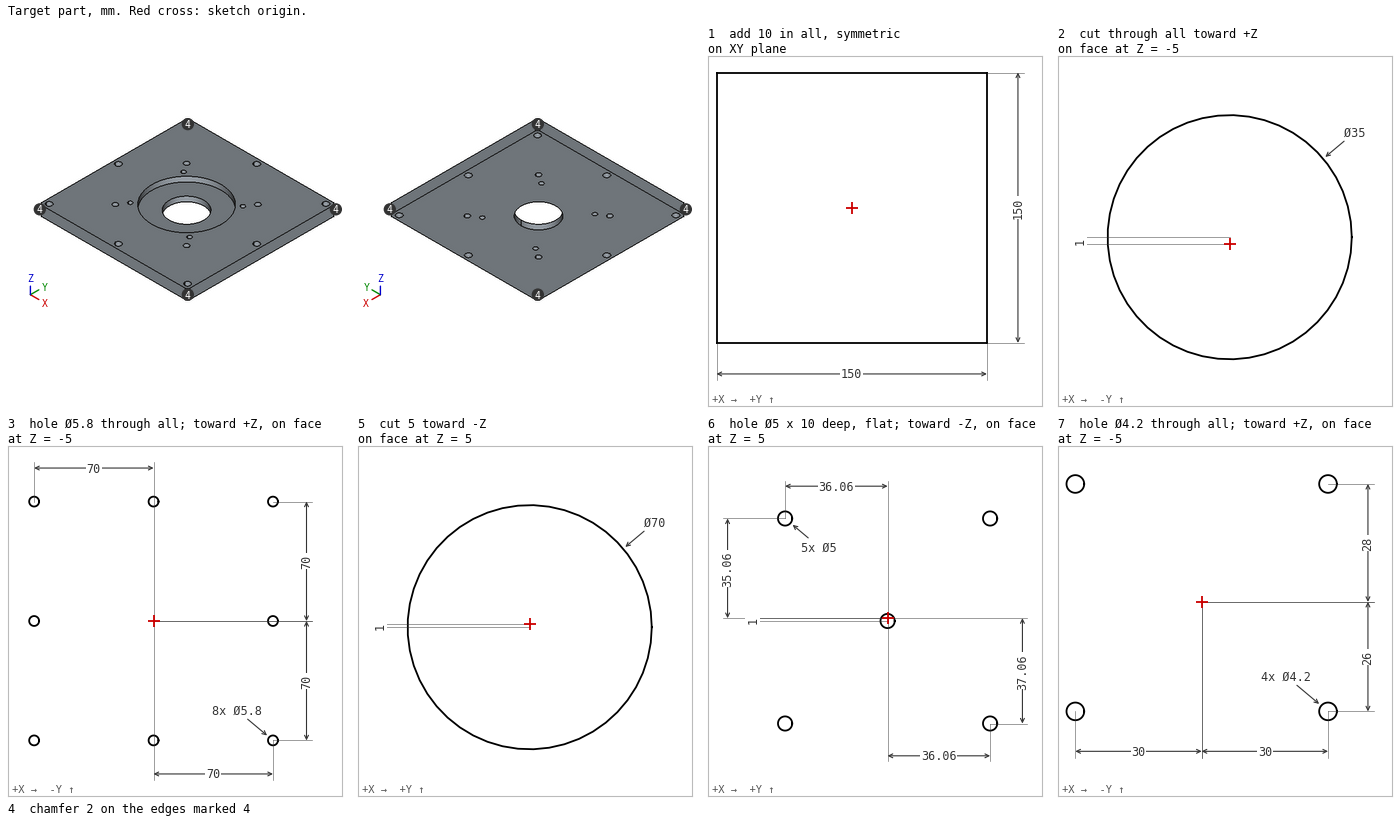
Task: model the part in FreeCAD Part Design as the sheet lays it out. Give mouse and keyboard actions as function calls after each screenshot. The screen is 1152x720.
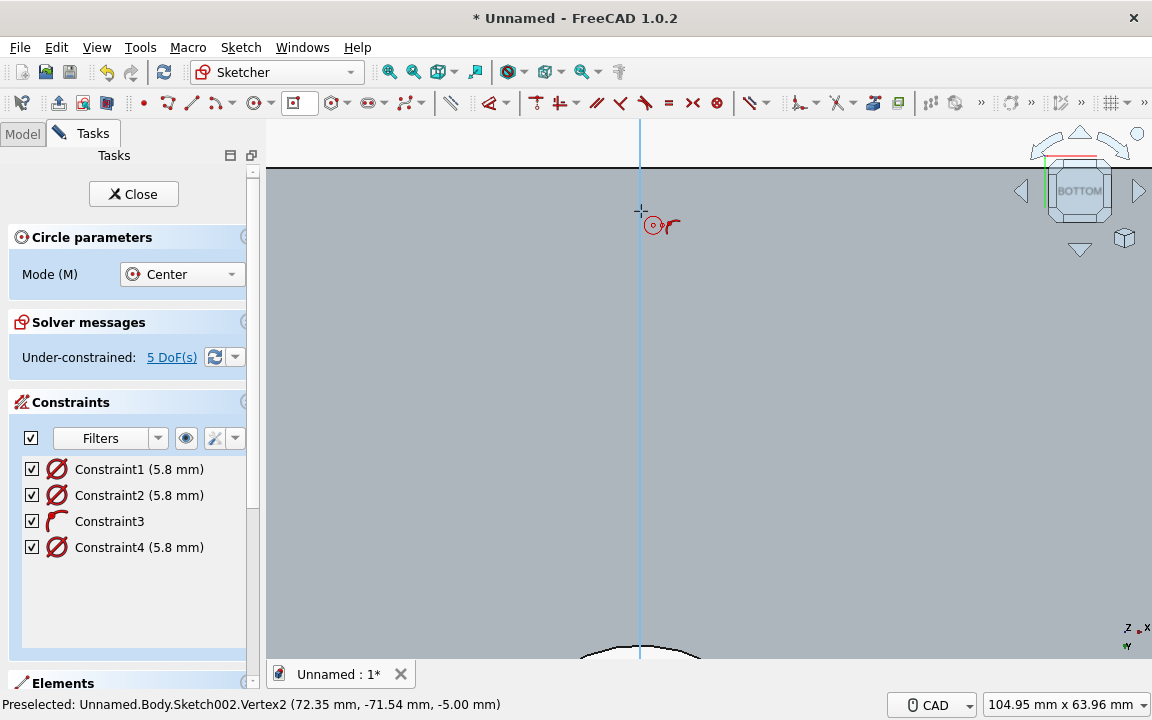
click(640, 211)
move(658, 193)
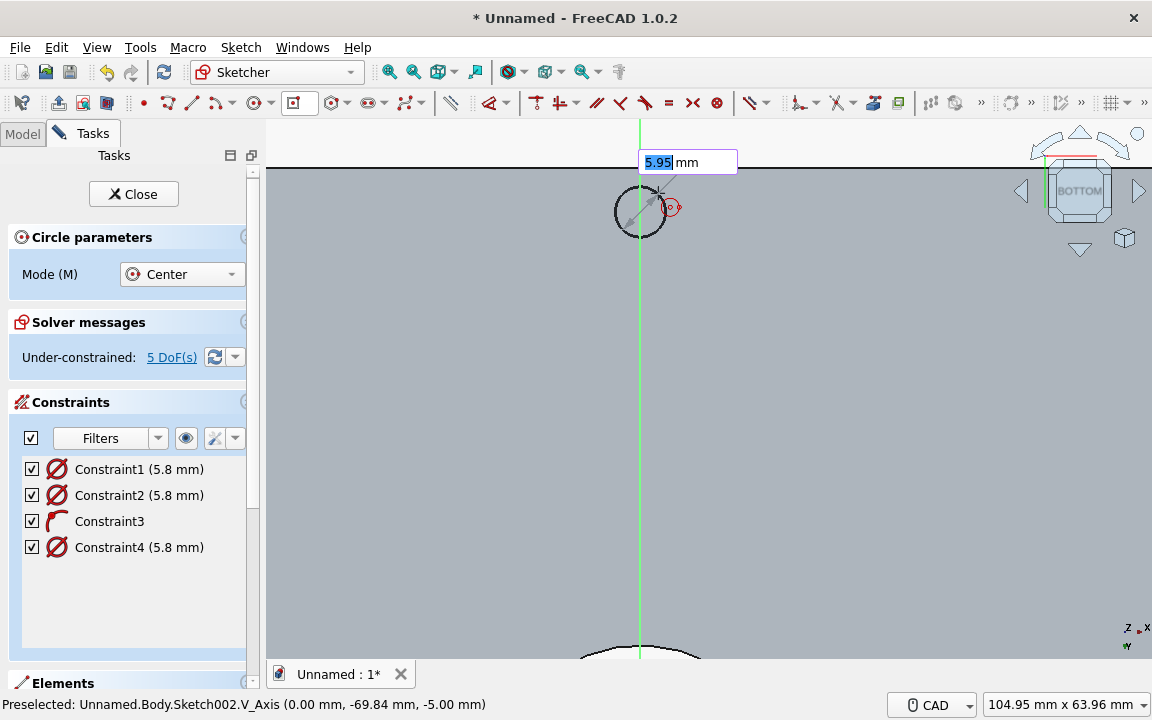
text(5.8)
key(Return)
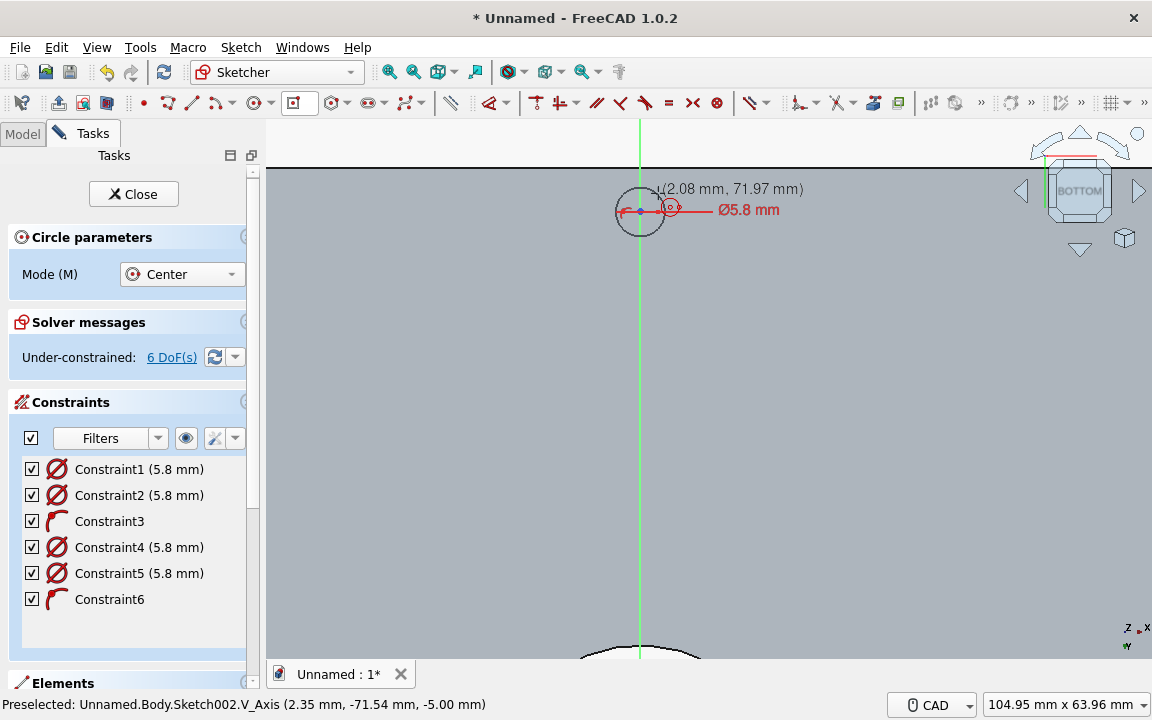
scroll(641, 211, down, 6)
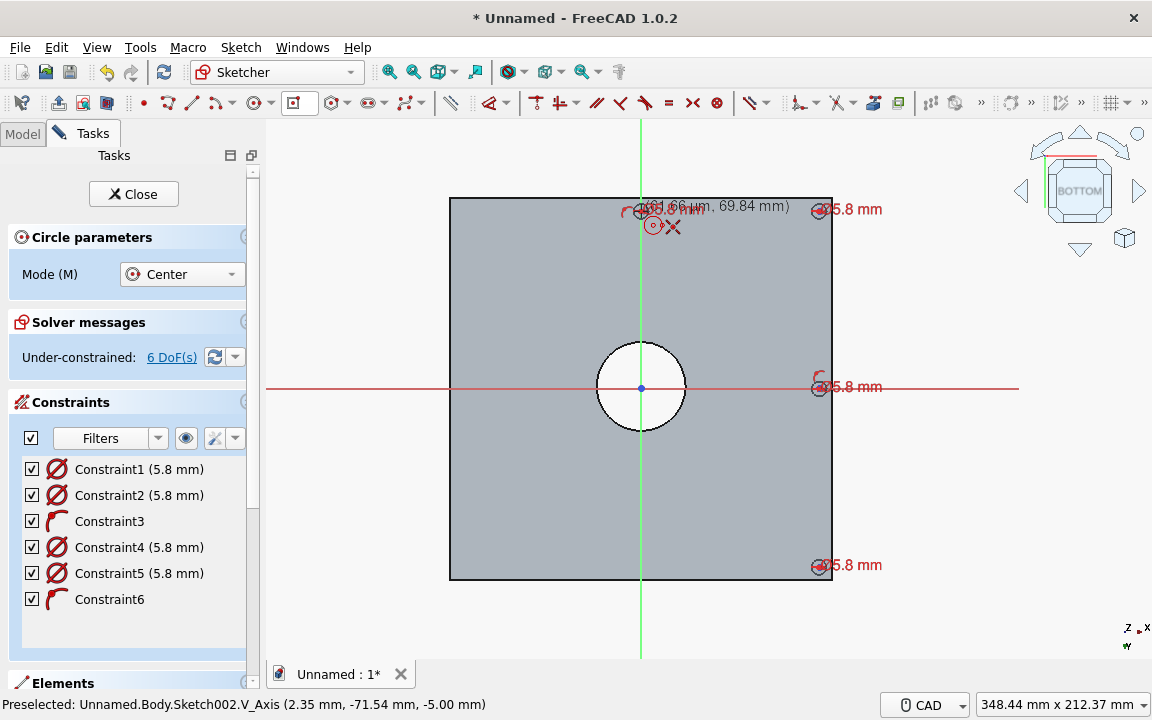
scroll(463, 211, up, 6)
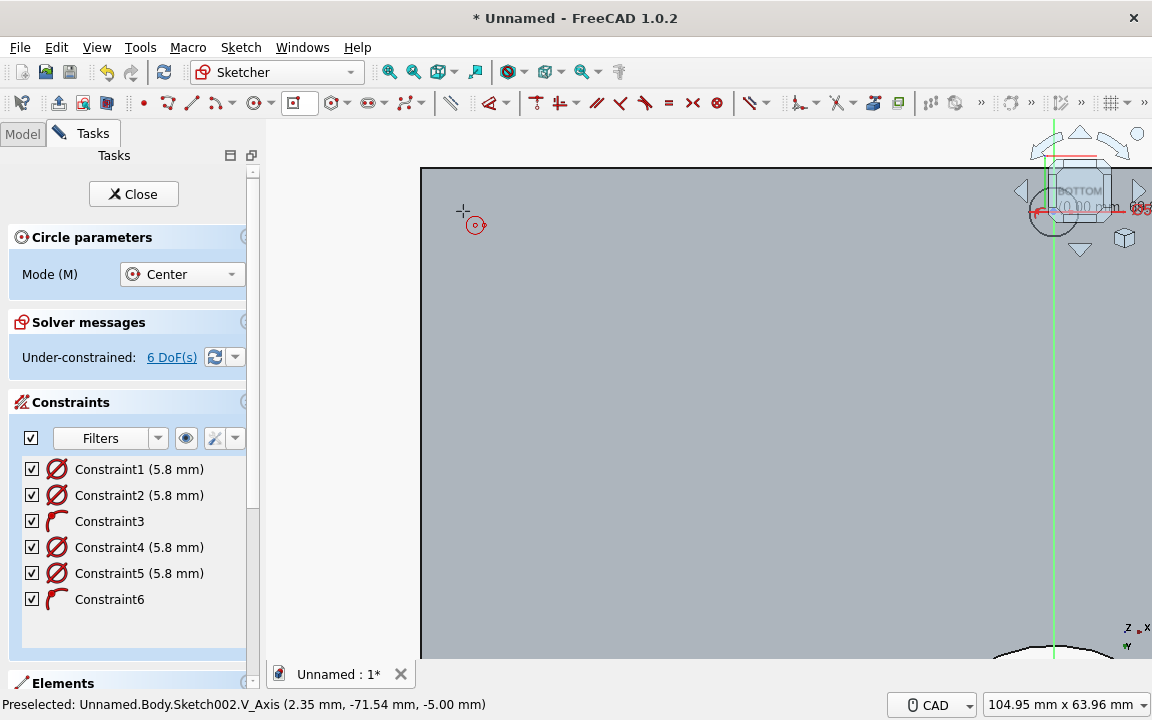
click(463, 211)
move(480, 193)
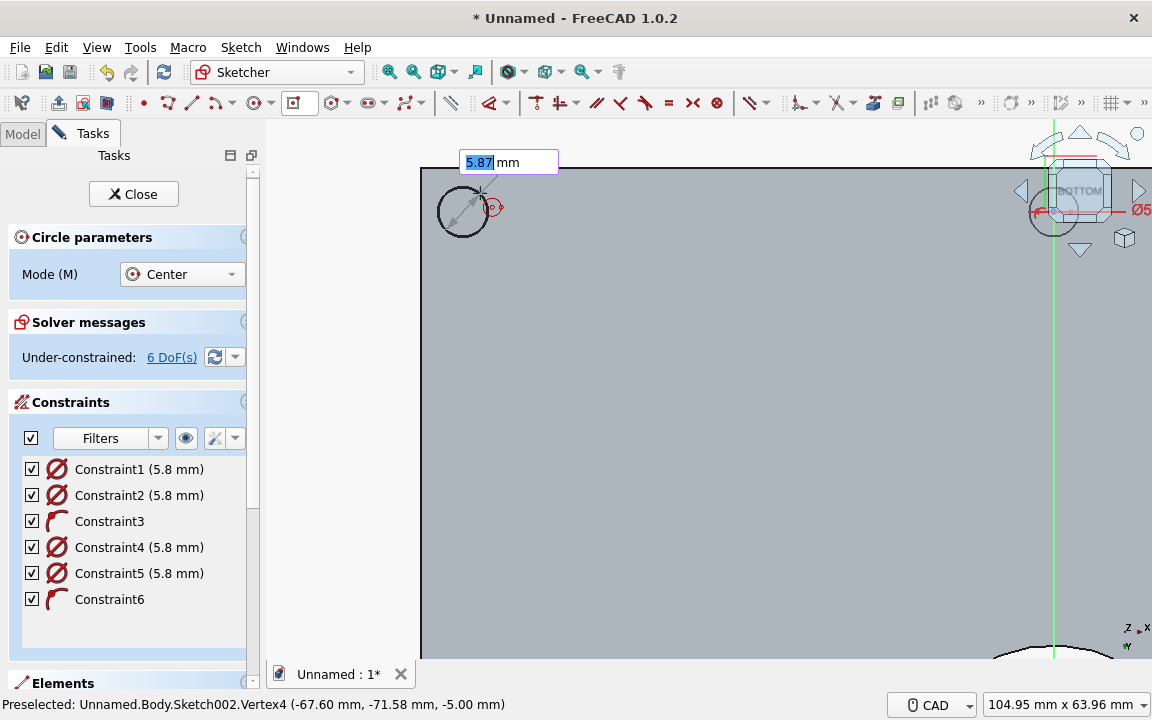
text(5.8)
key(Return)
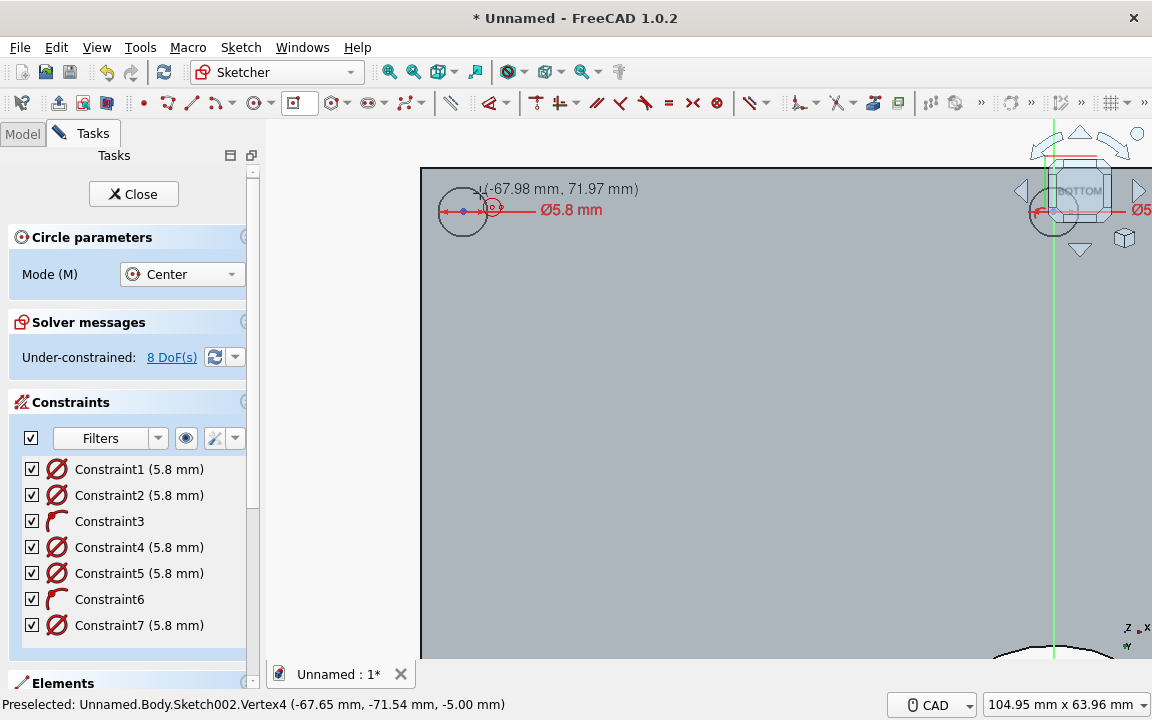
scroll(462, 211, down, 6)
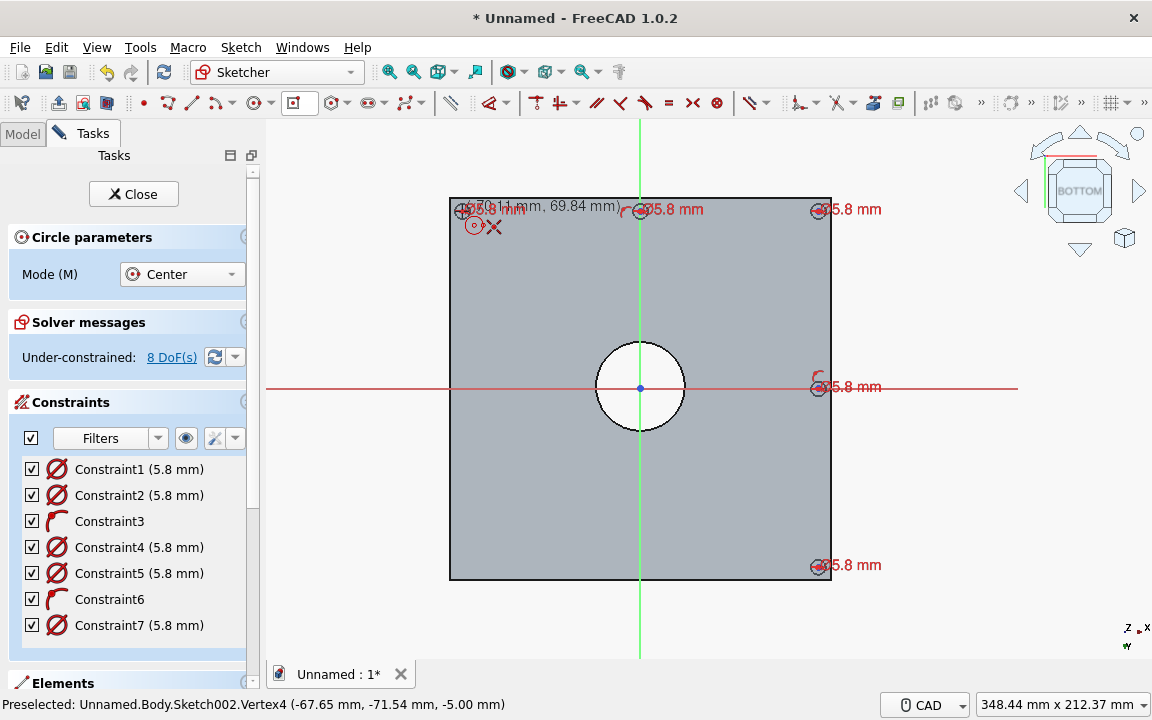
scroll(462, 389, up, 6)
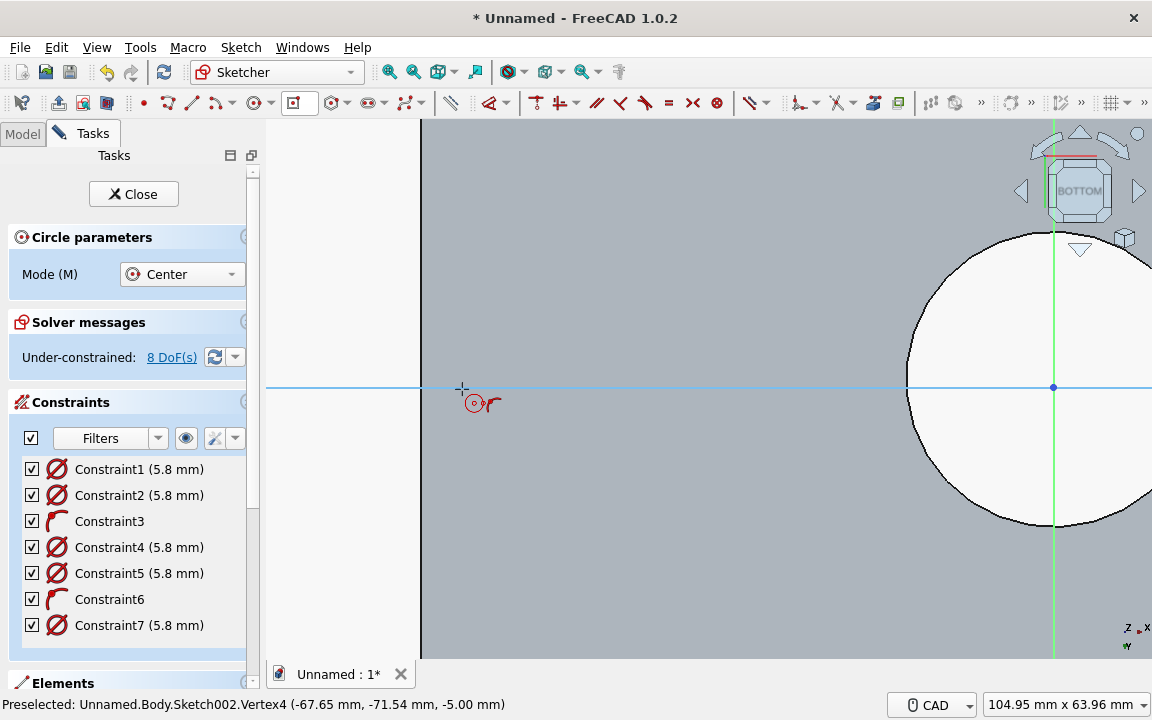
click(463, 388)
move(480, 371)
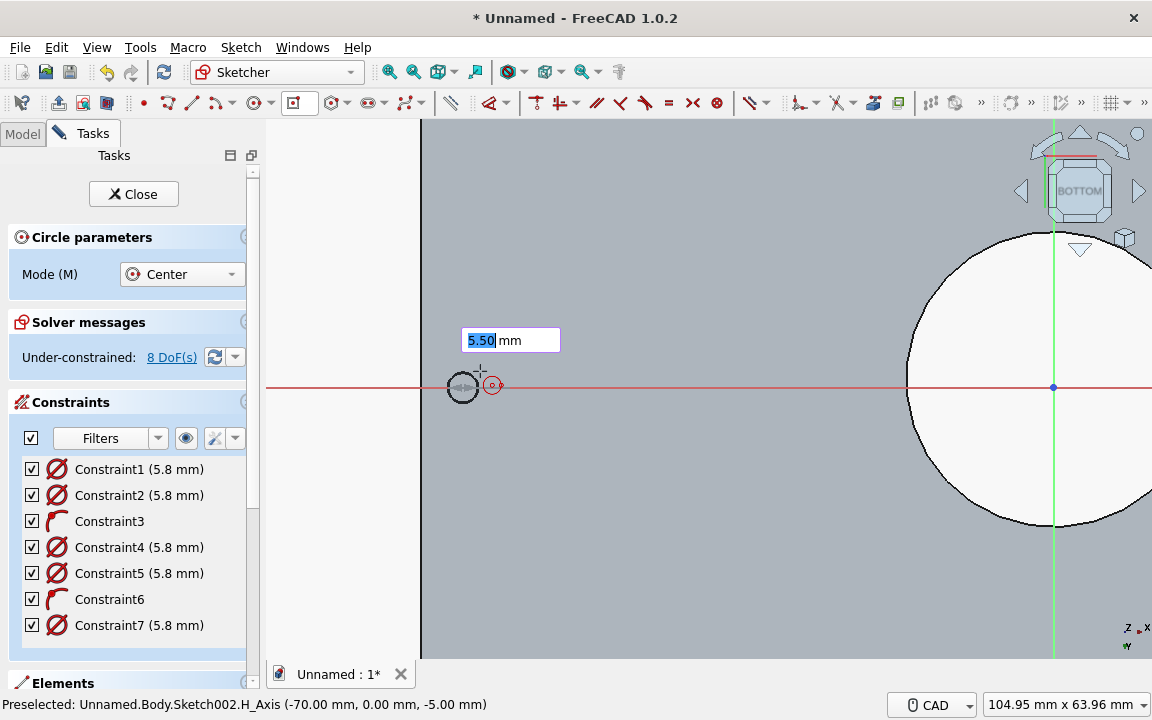
text(5.8)
key(Return)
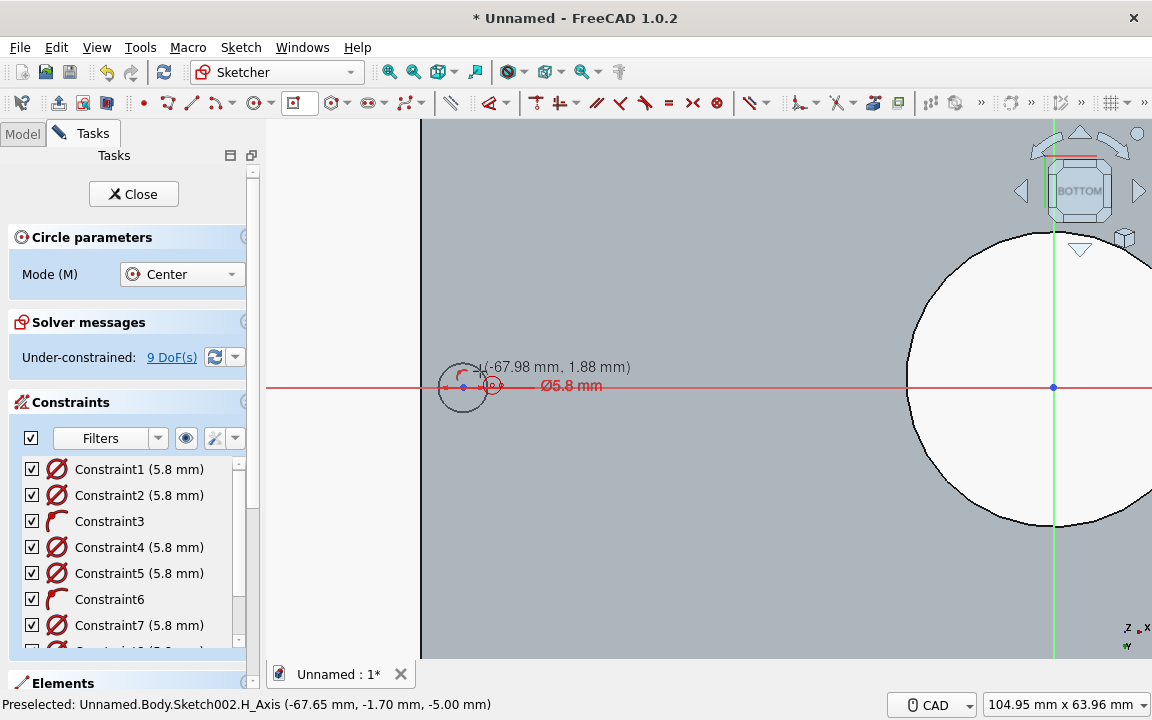
scroll(462, 390, down, 6)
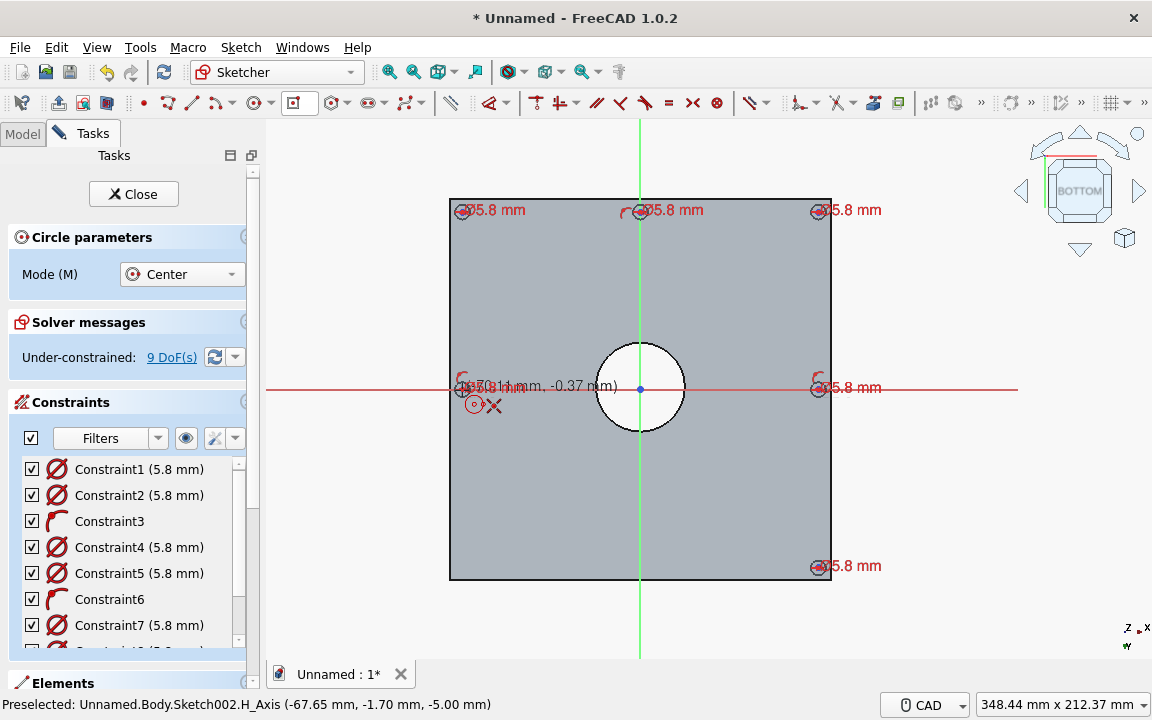
scroll(462, 568, up, 6)